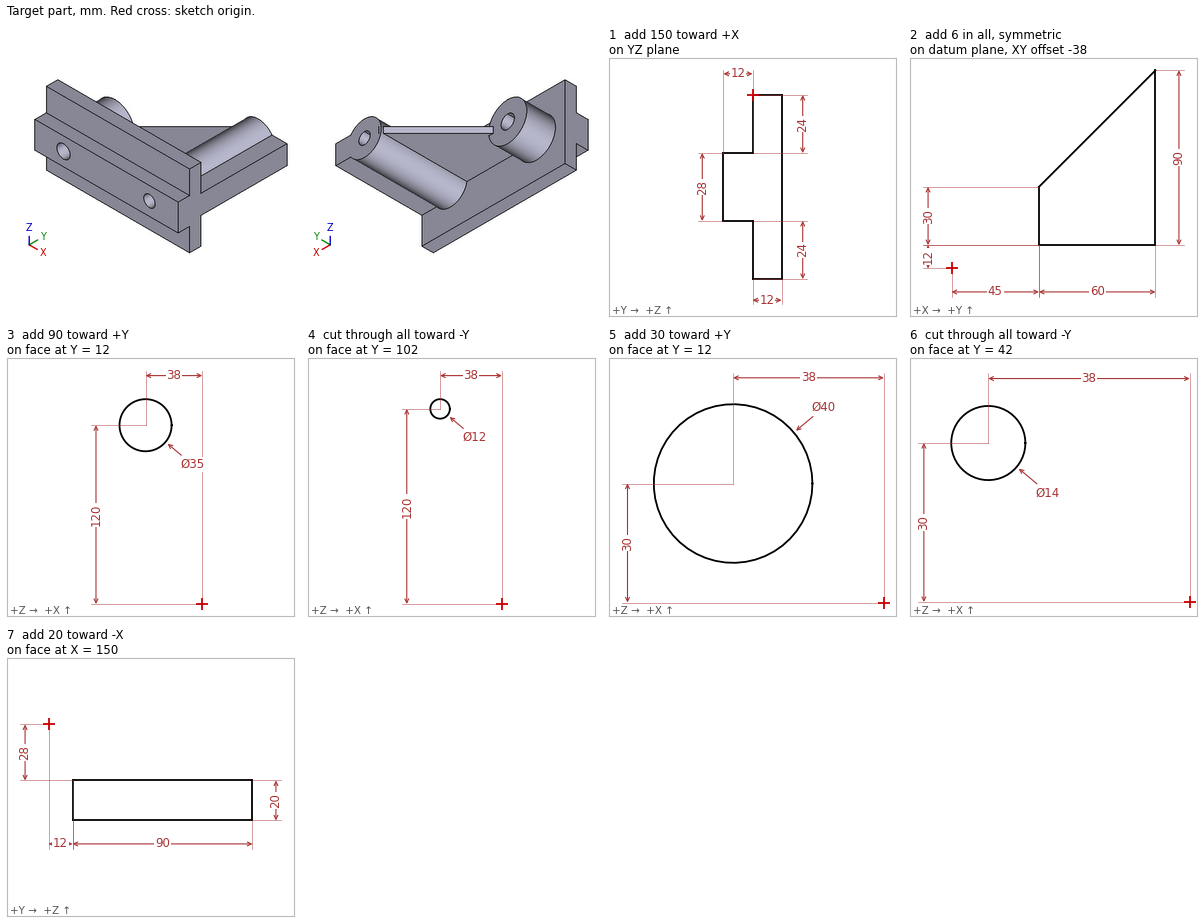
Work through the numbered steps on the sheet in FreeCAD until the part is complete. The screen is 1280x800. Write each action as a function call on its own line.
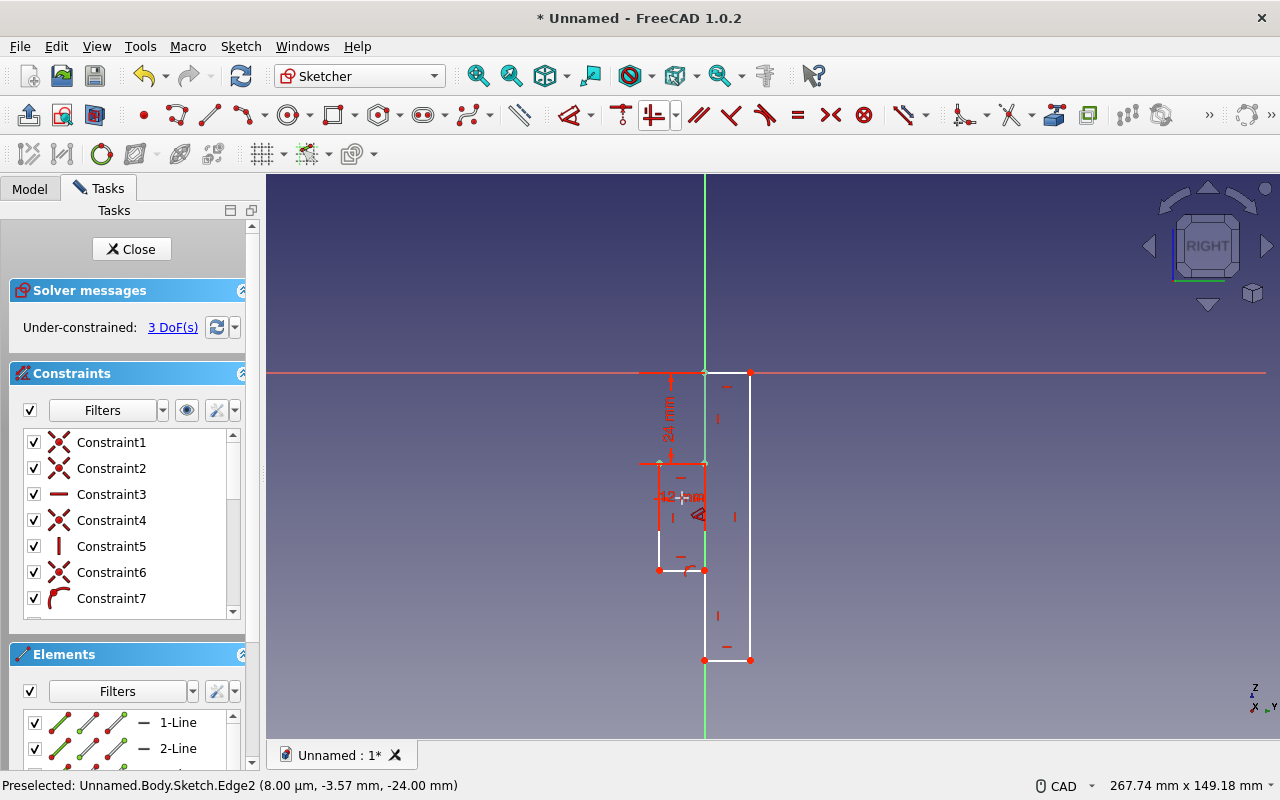
click(659, 496)
click(625, 542)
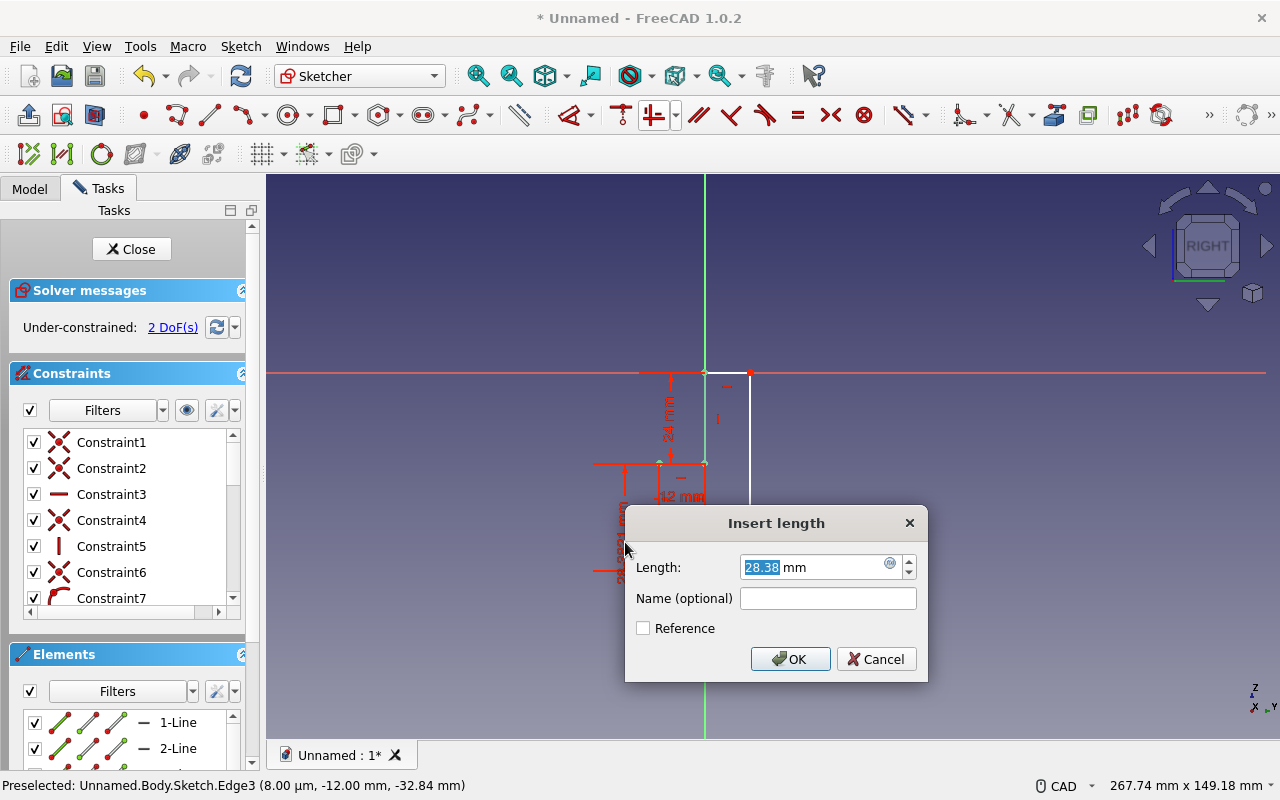
text(28)
key(Return)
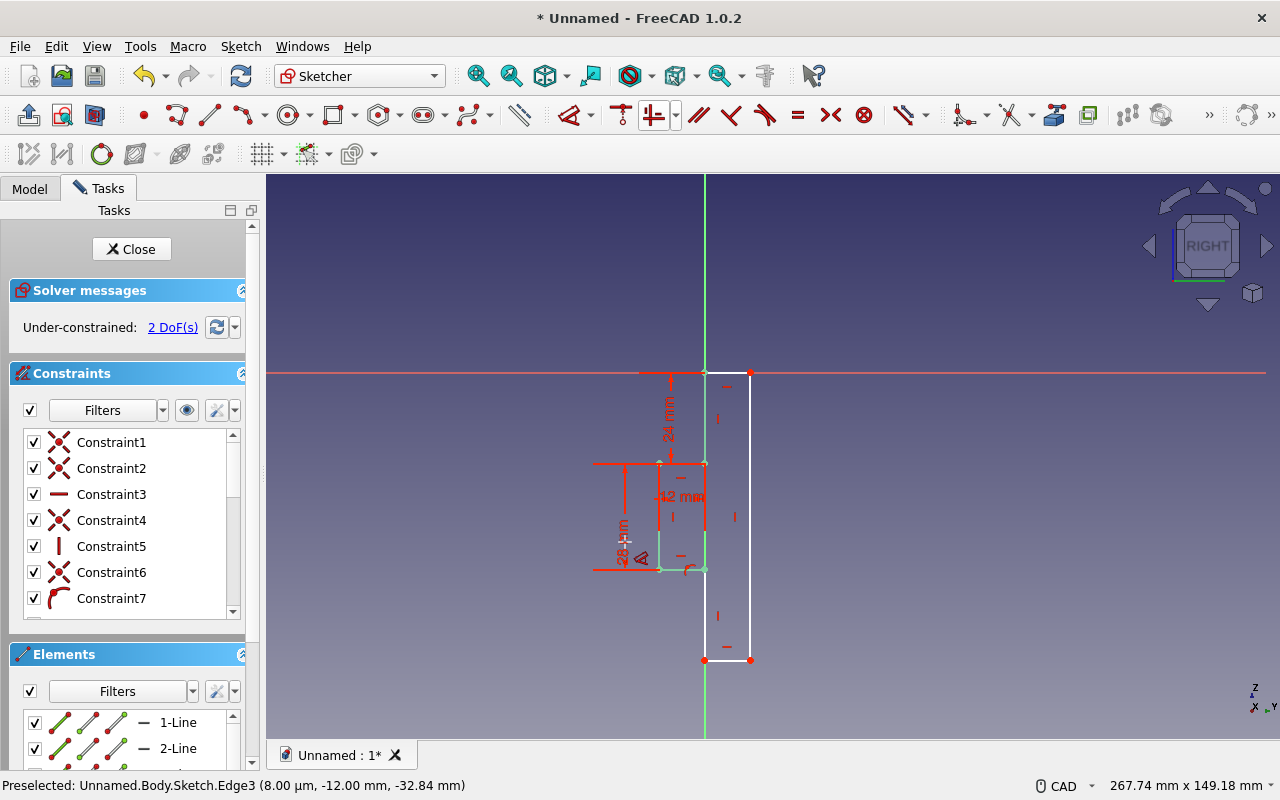
click(705, 597)
click(671, 615)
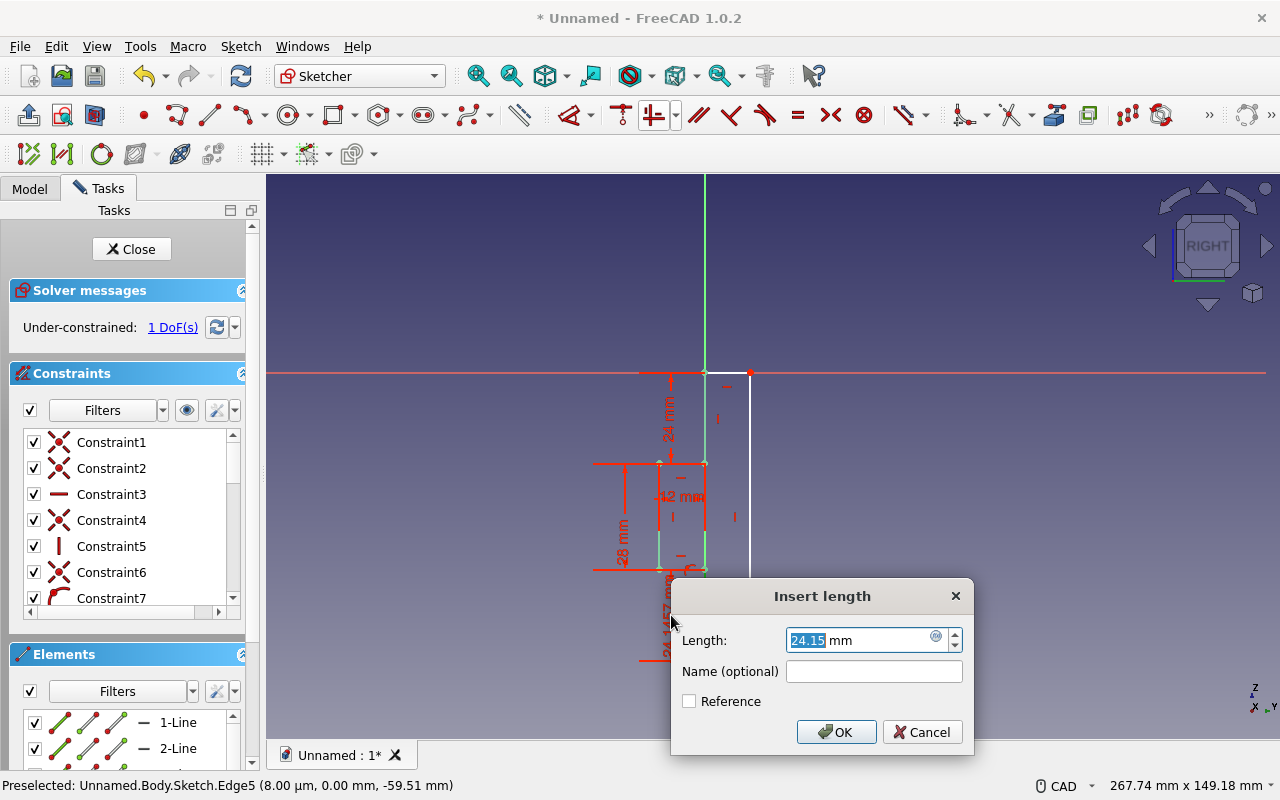
text(24)
key(Return)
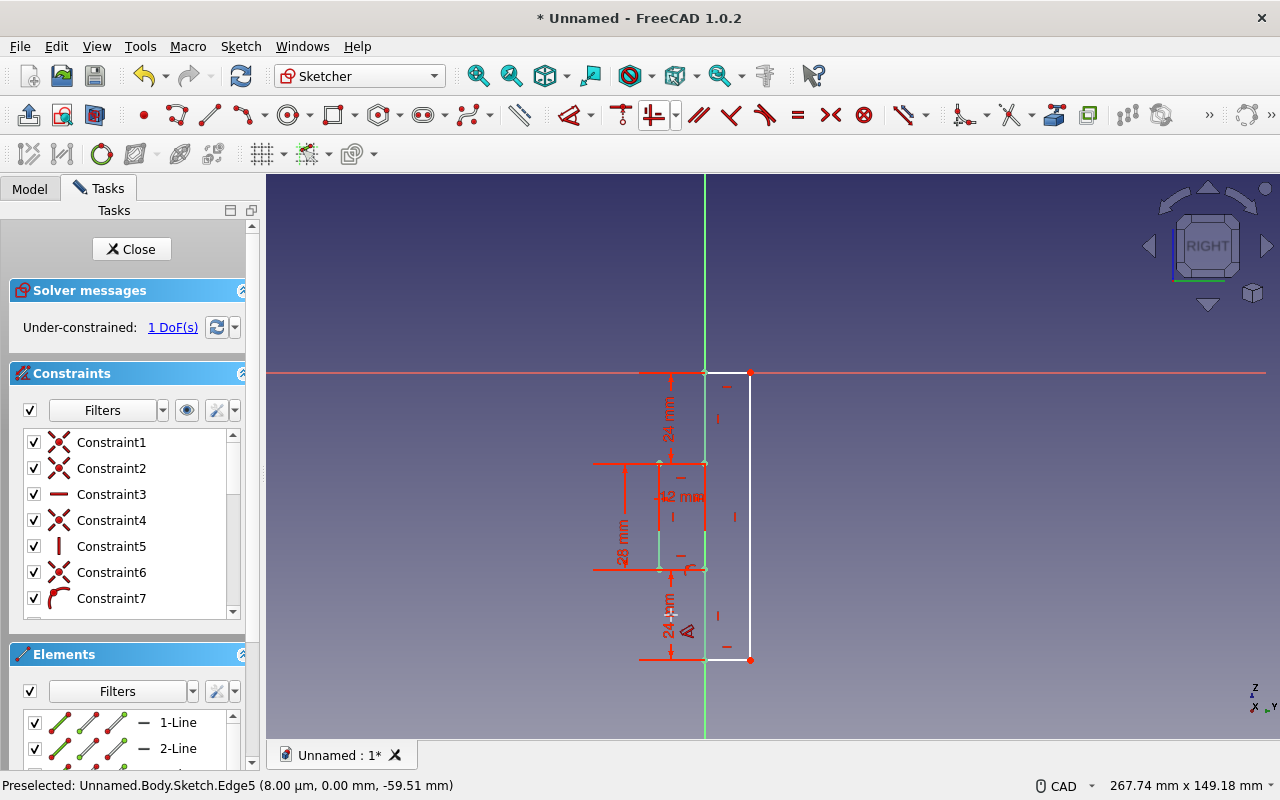
click(718, 660)
click(727, 694)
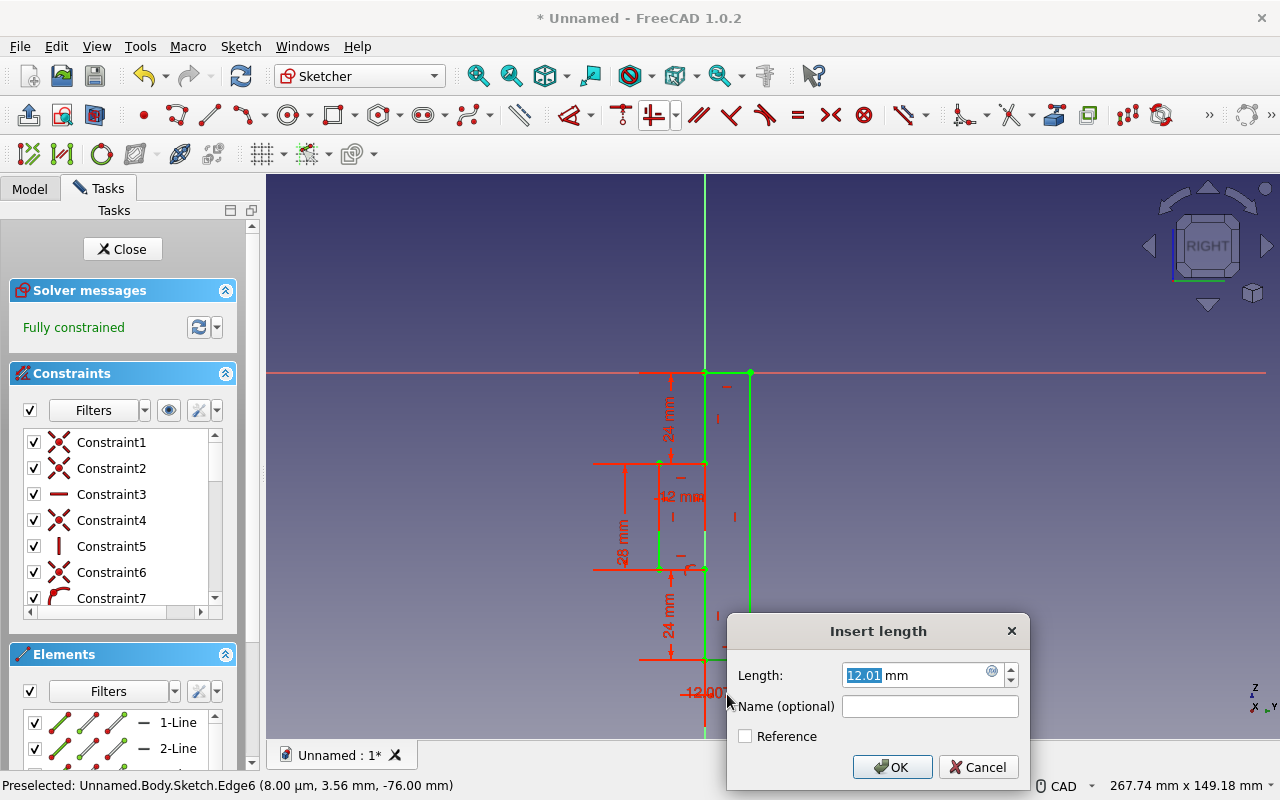
text(12)
key(Return)
key(Escape)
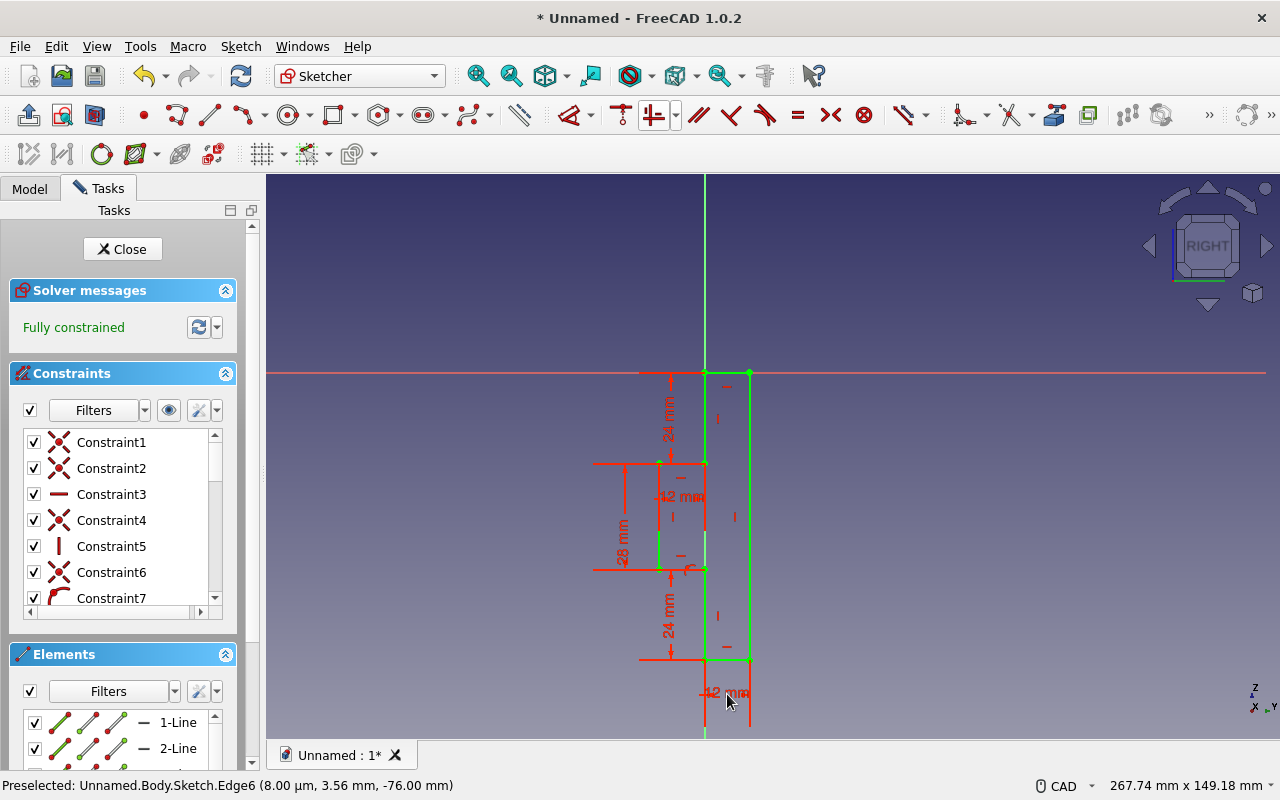
click(123, 249)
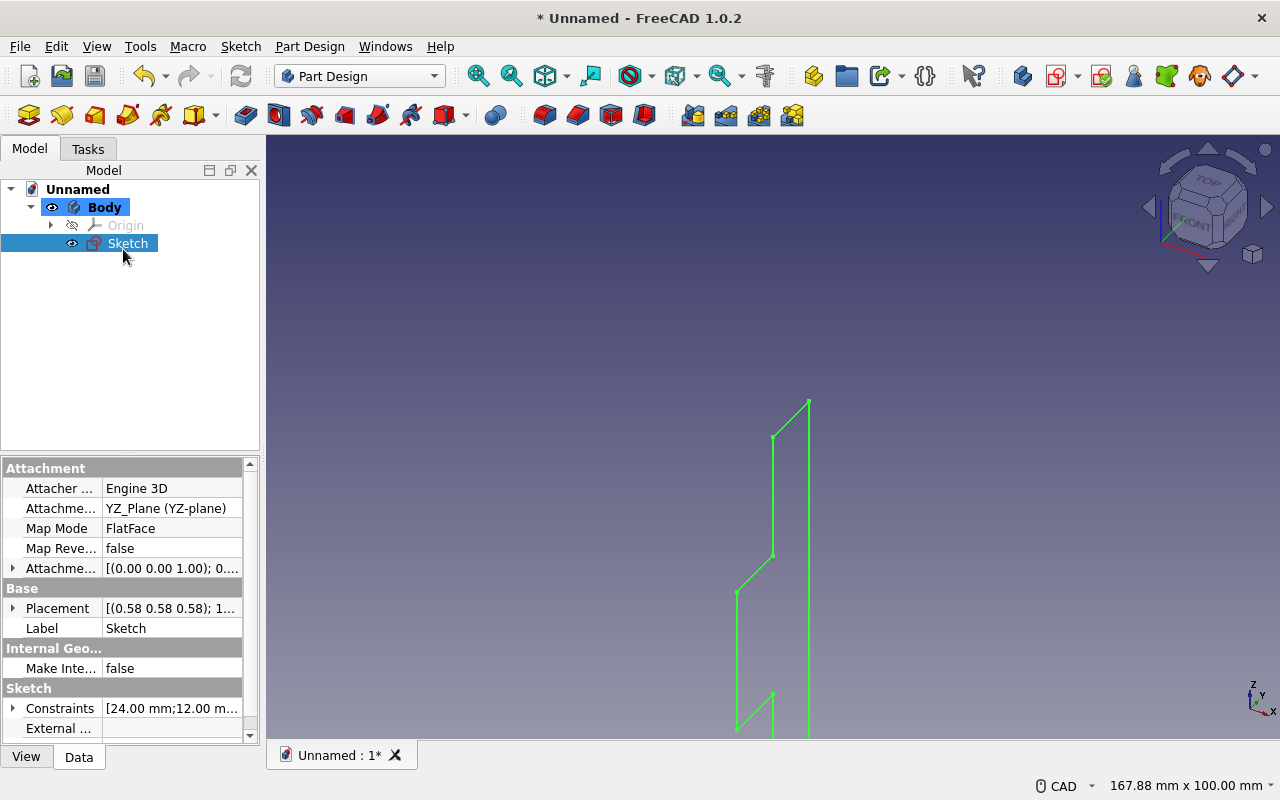
click(29, 116)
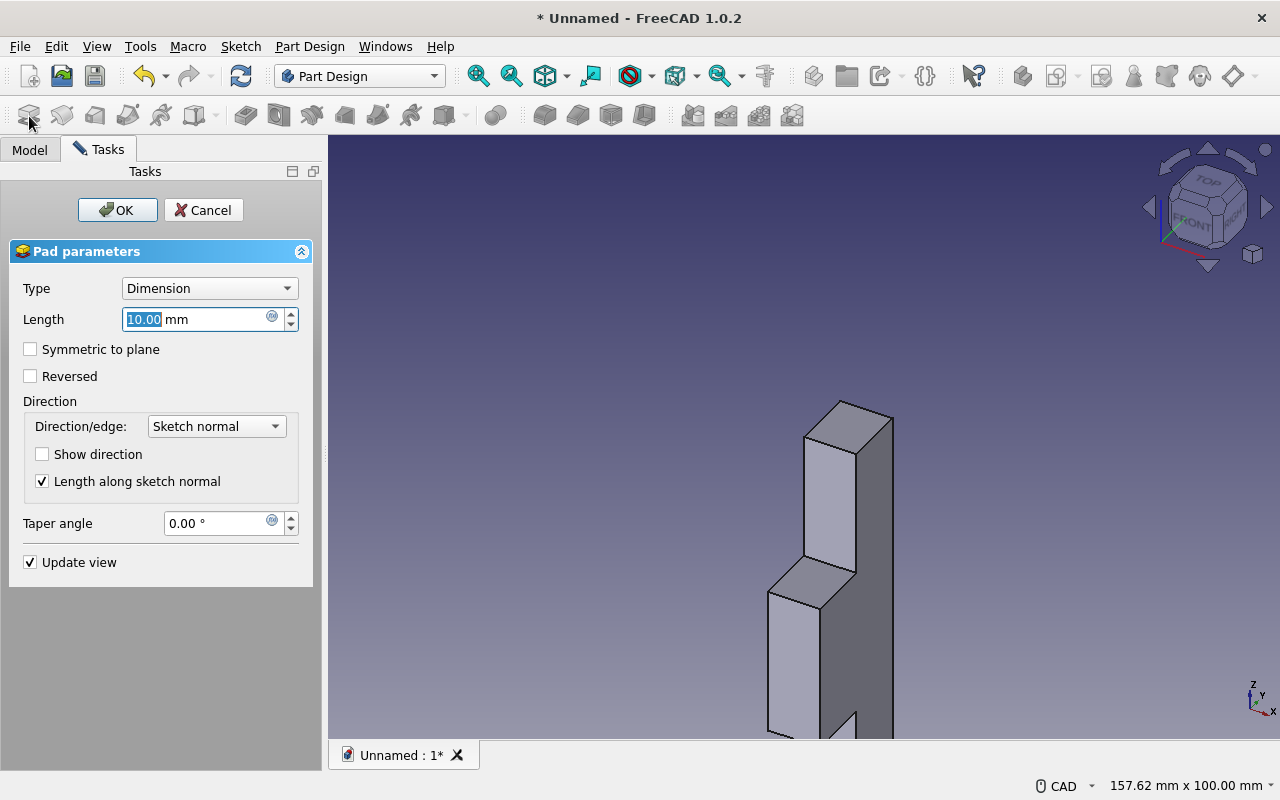
text(150)
key(Tab)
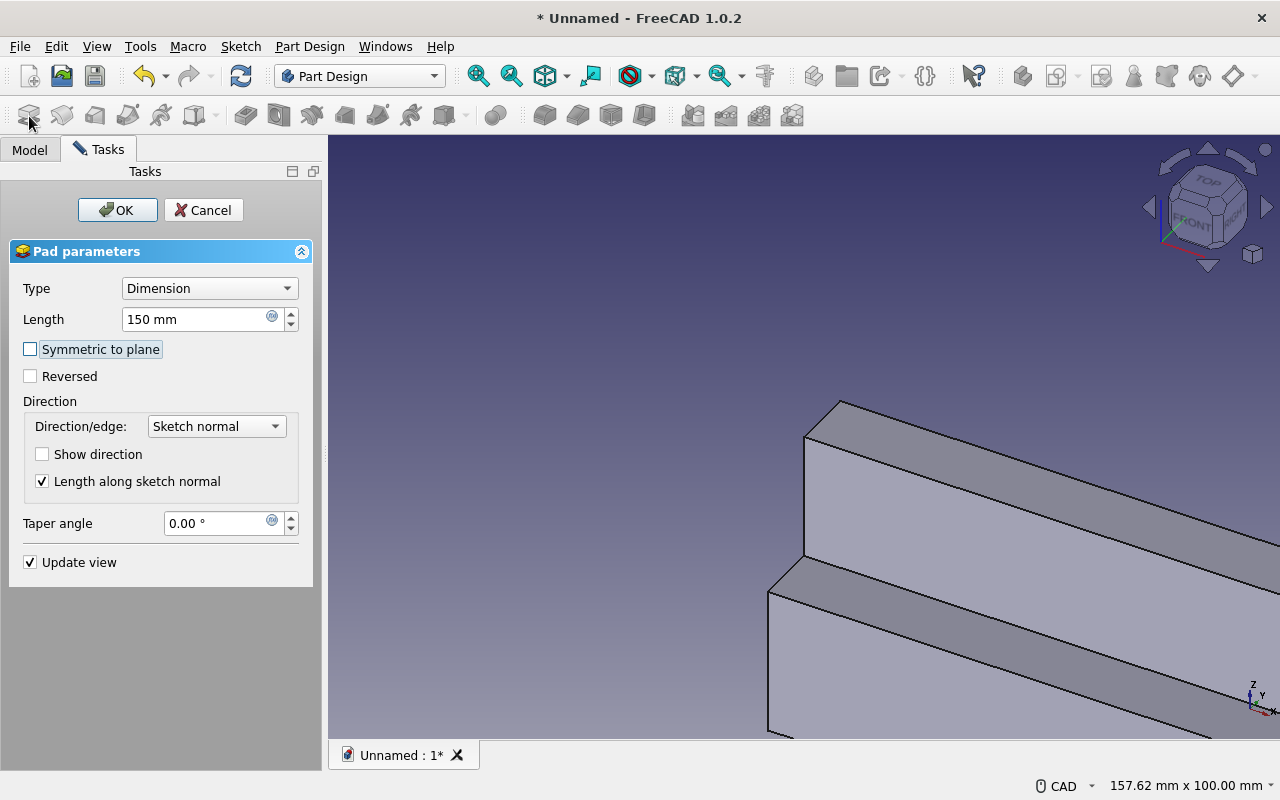
click(118, 210)